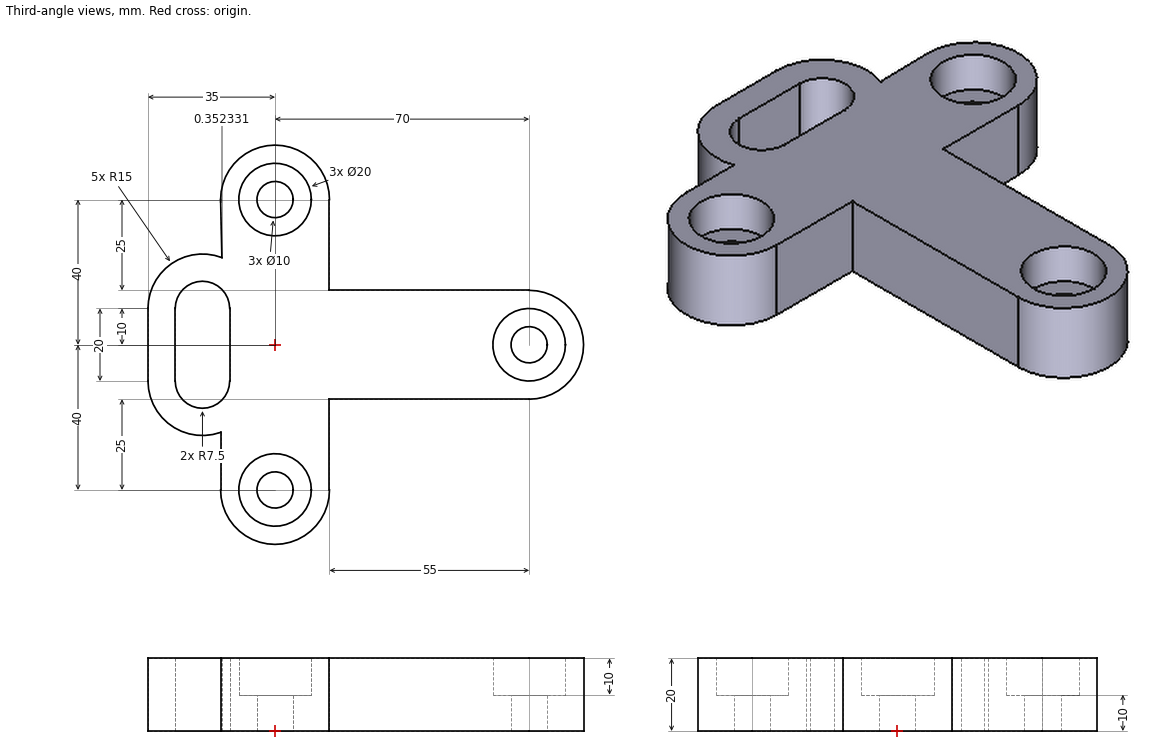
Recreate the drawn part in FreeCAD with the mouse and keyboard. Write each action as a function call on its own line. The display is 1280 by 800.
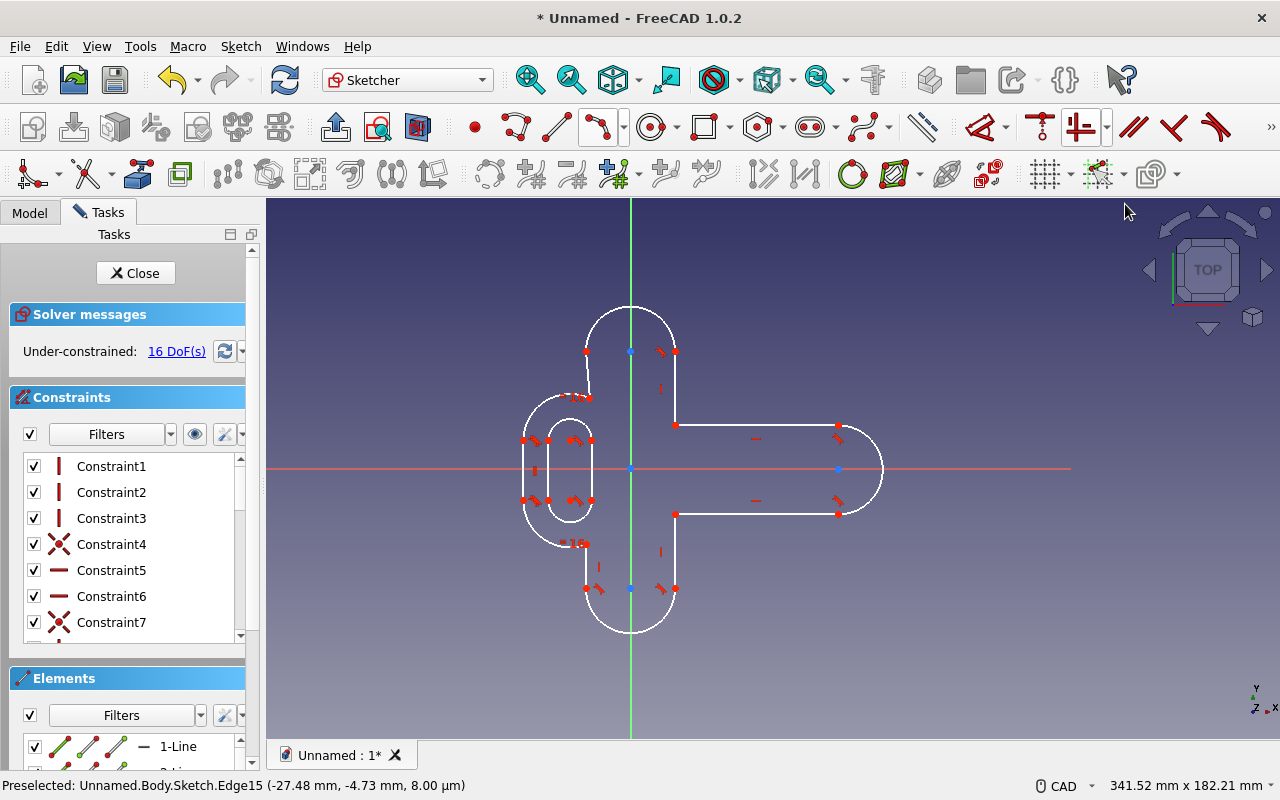
click(531, 526)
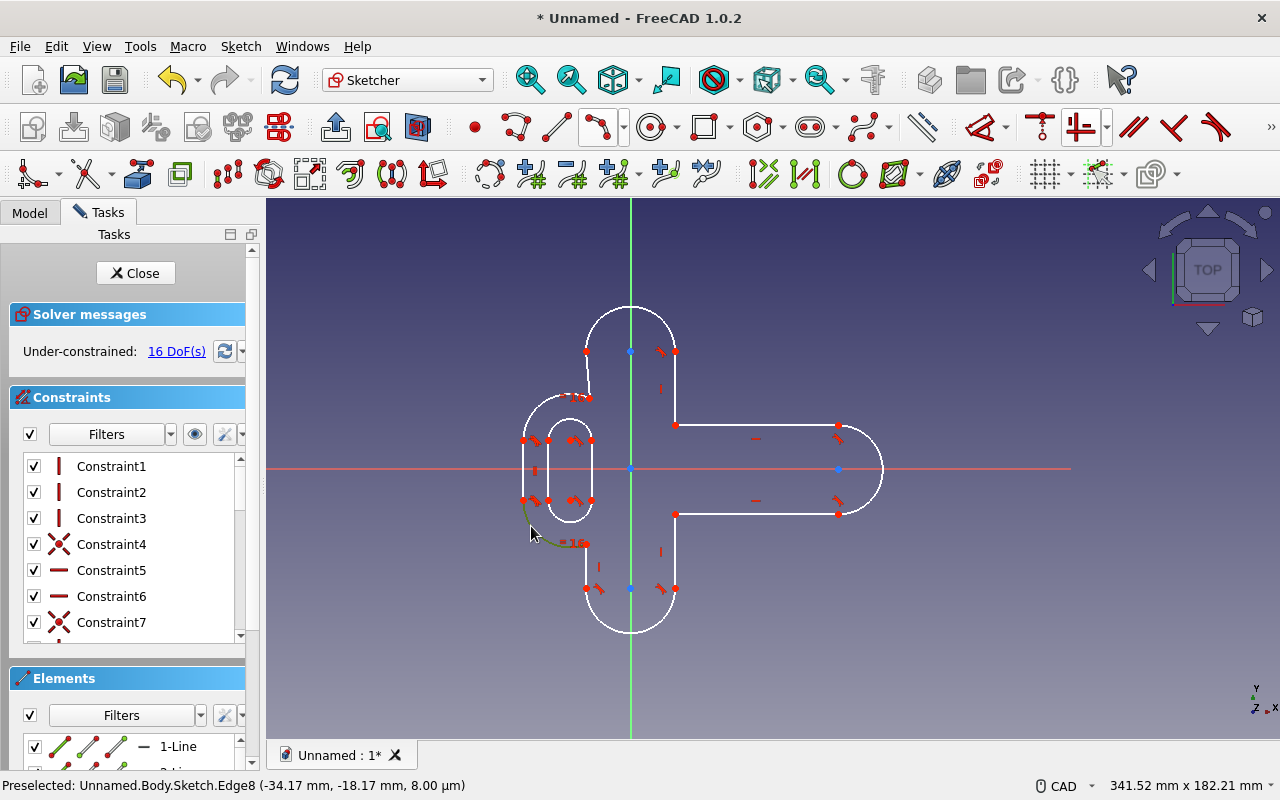
click(604, 625)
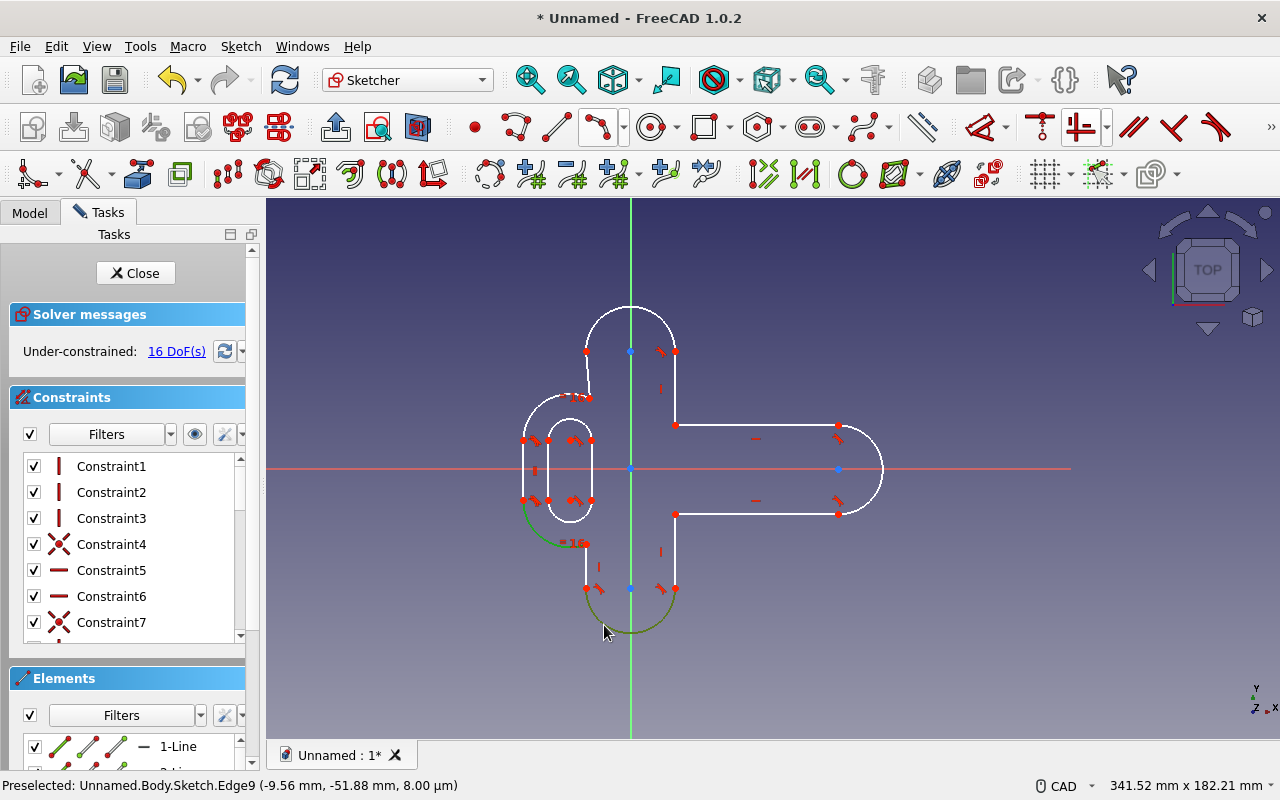
click(874, 496)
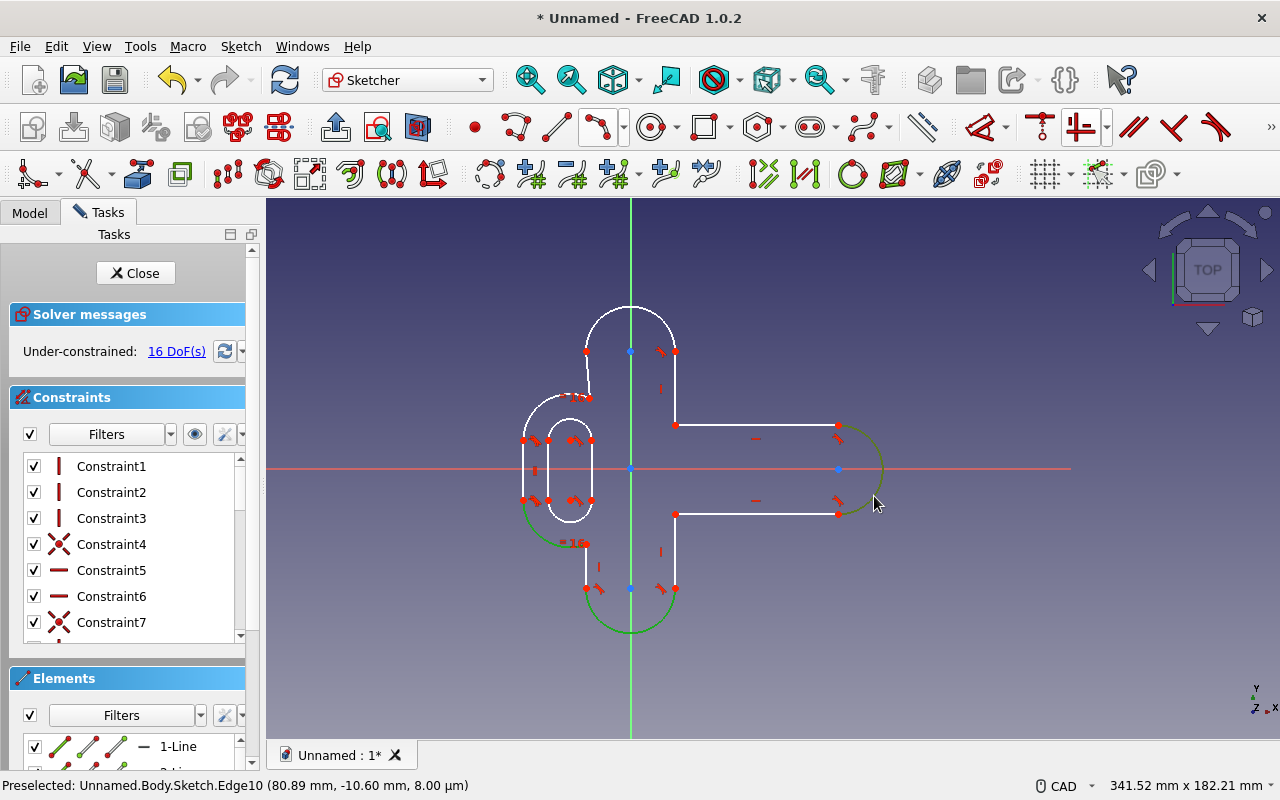
click(657, 315)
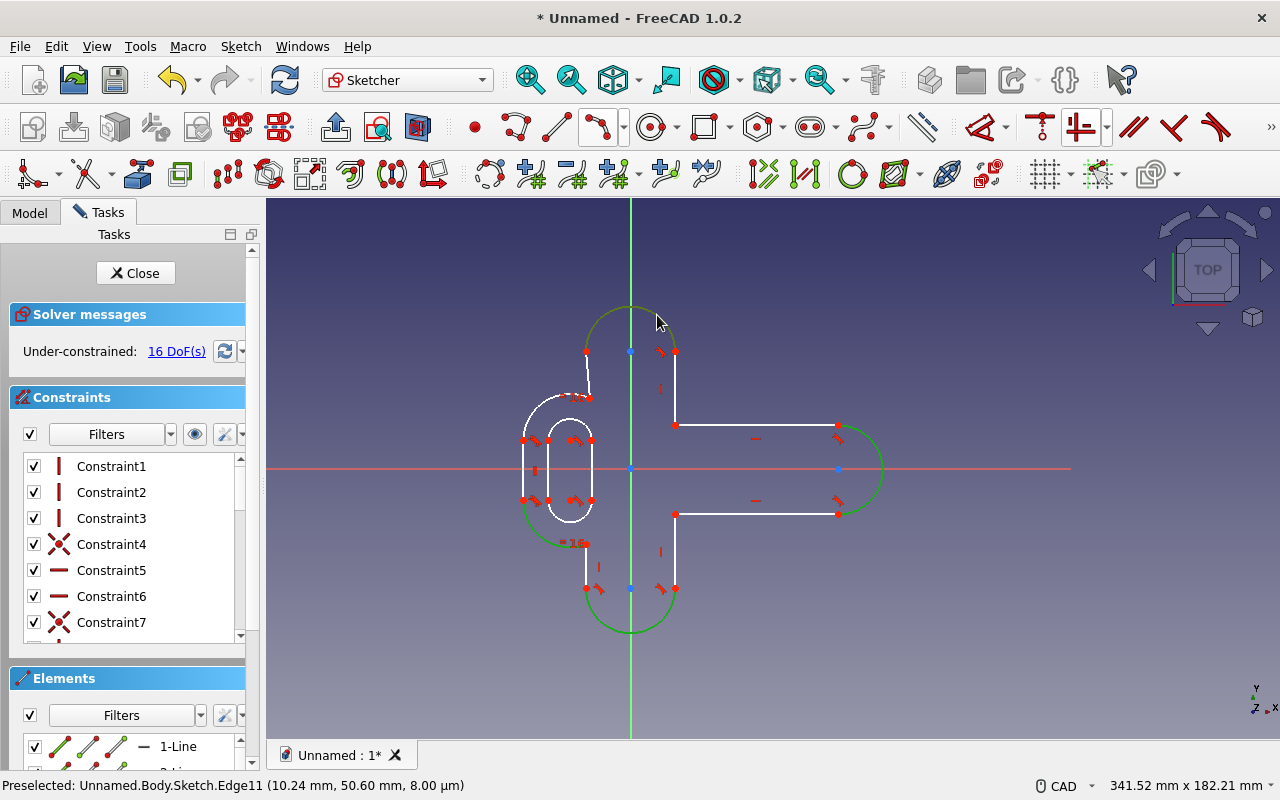
key(e)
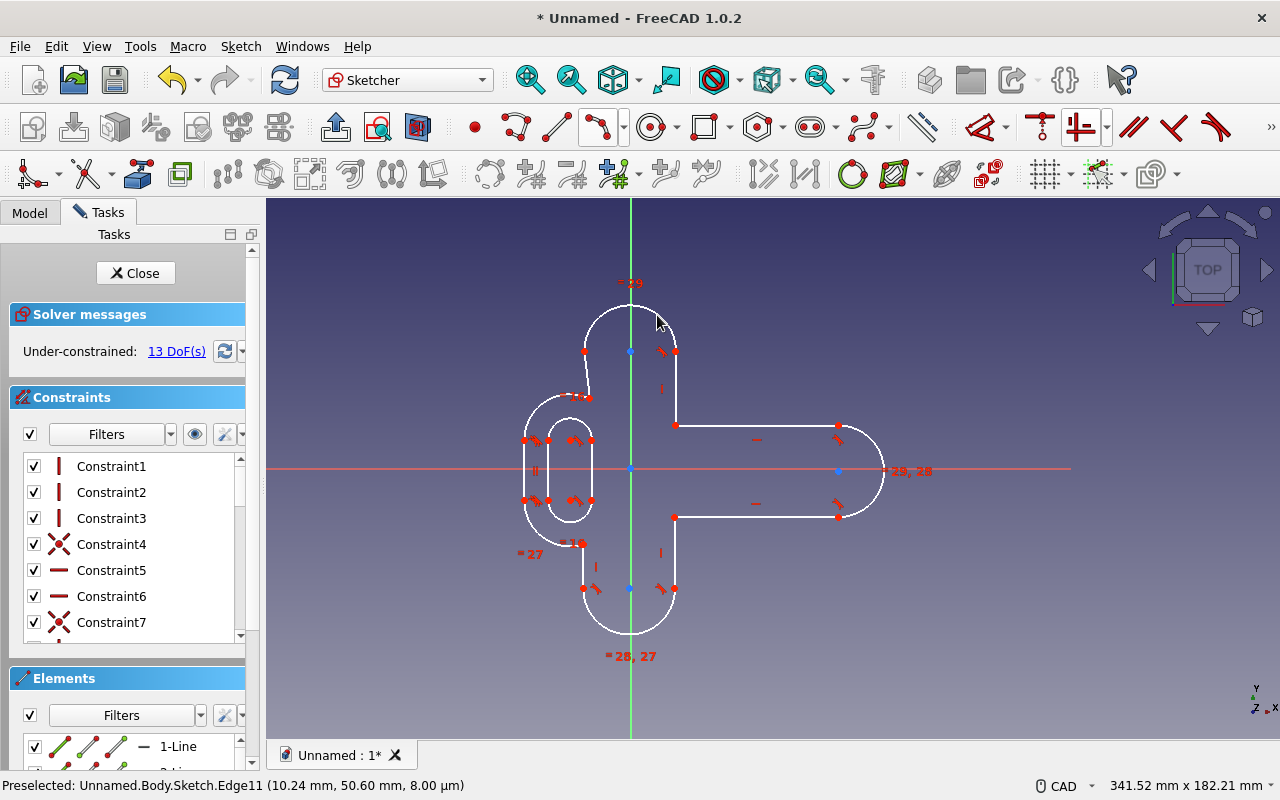
click(629, 589)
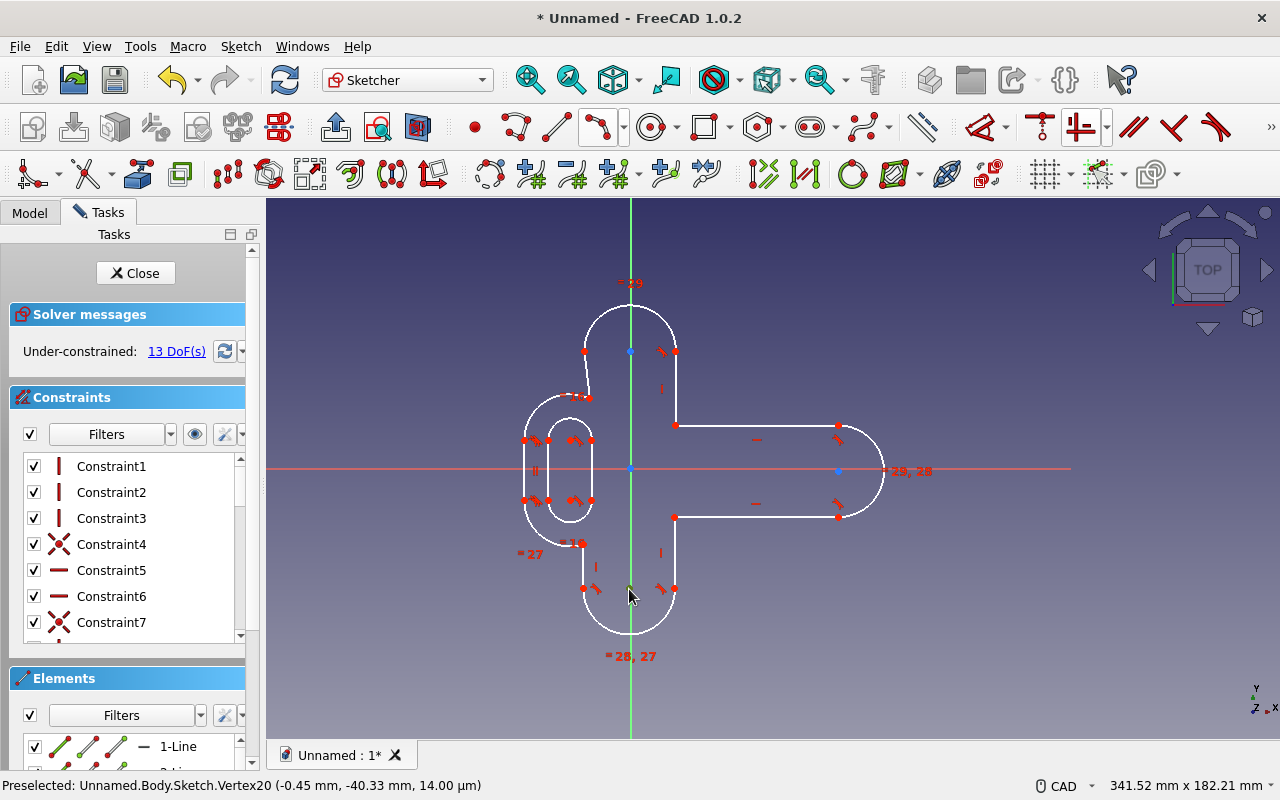
click(631, 676)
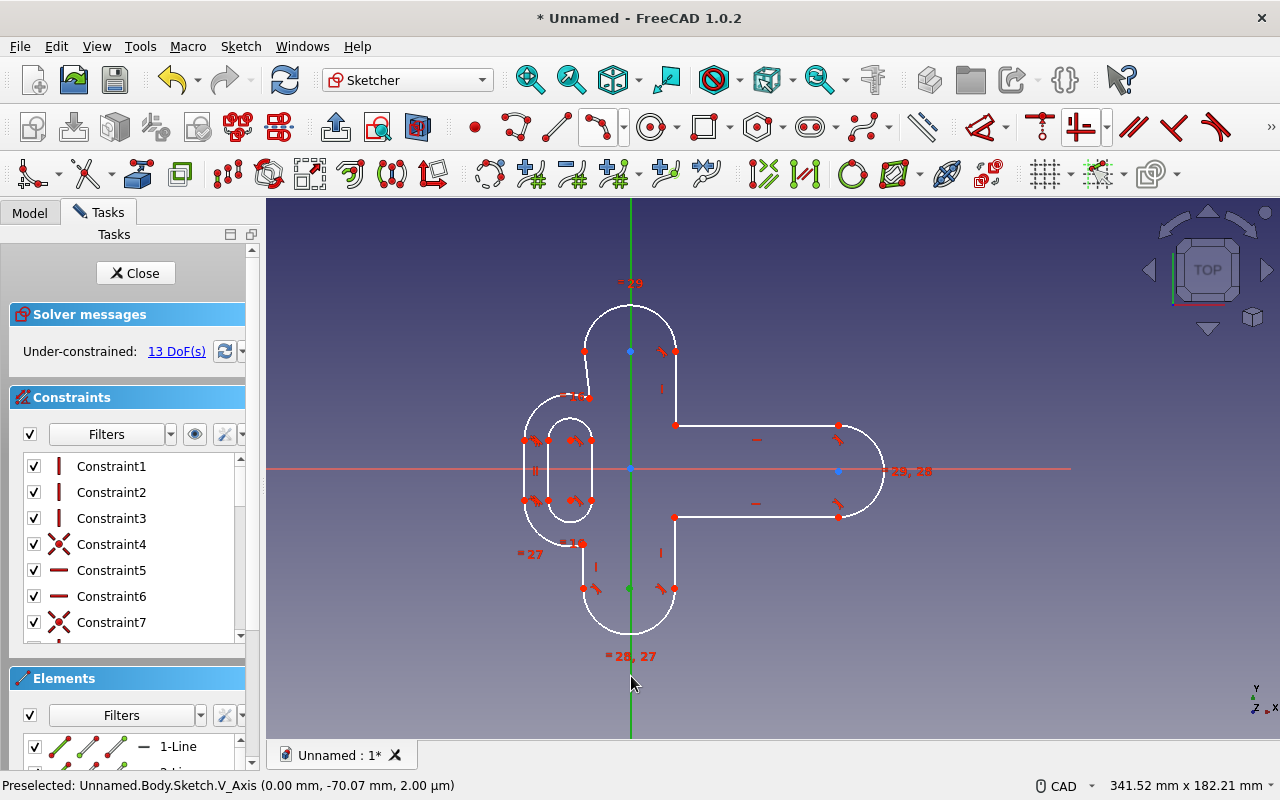
click(1040, 128)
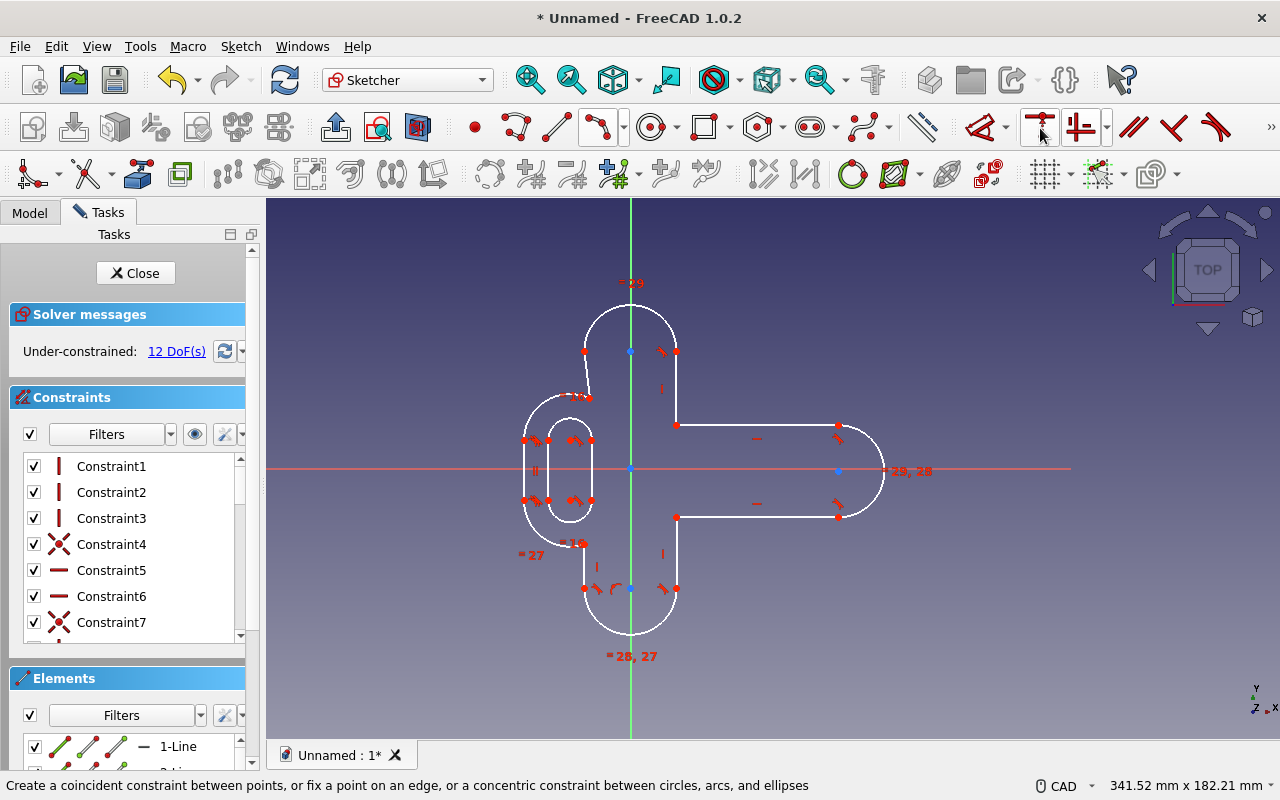
click(838, 471)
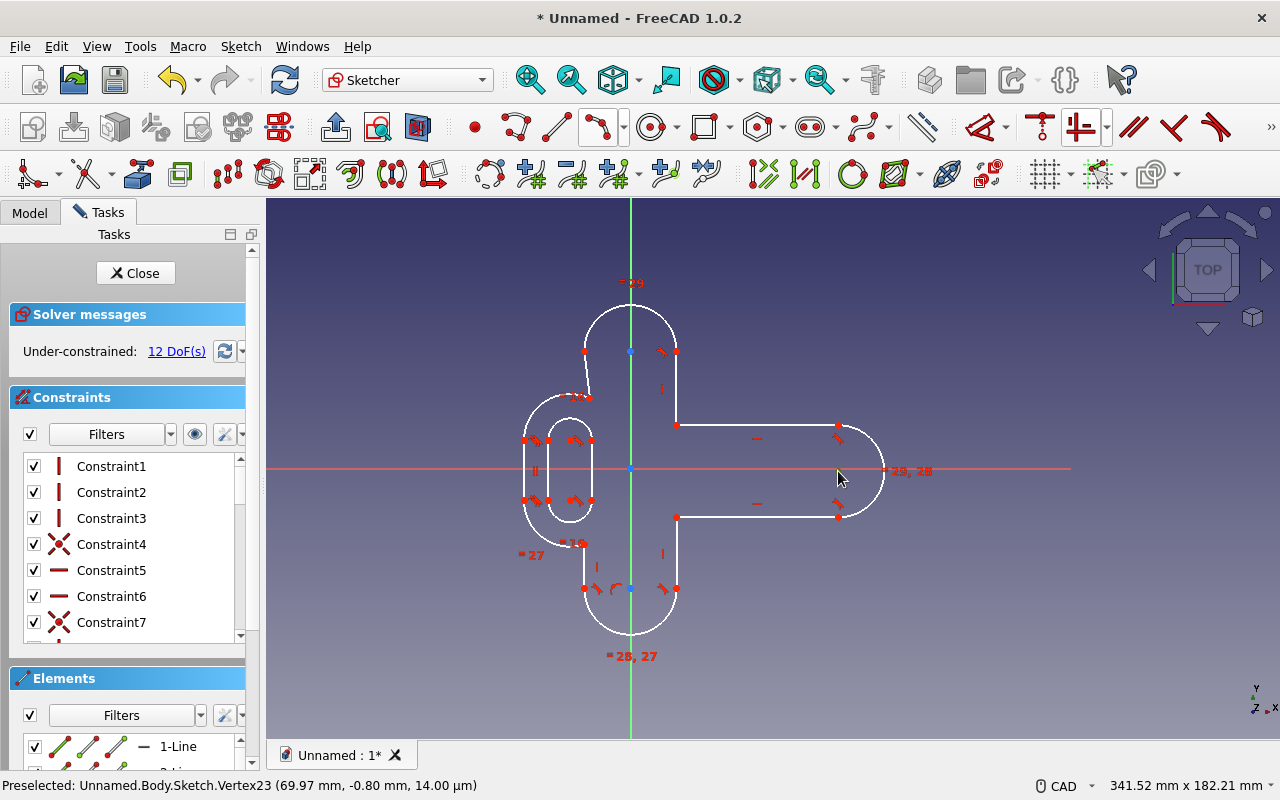
click(353, 469)